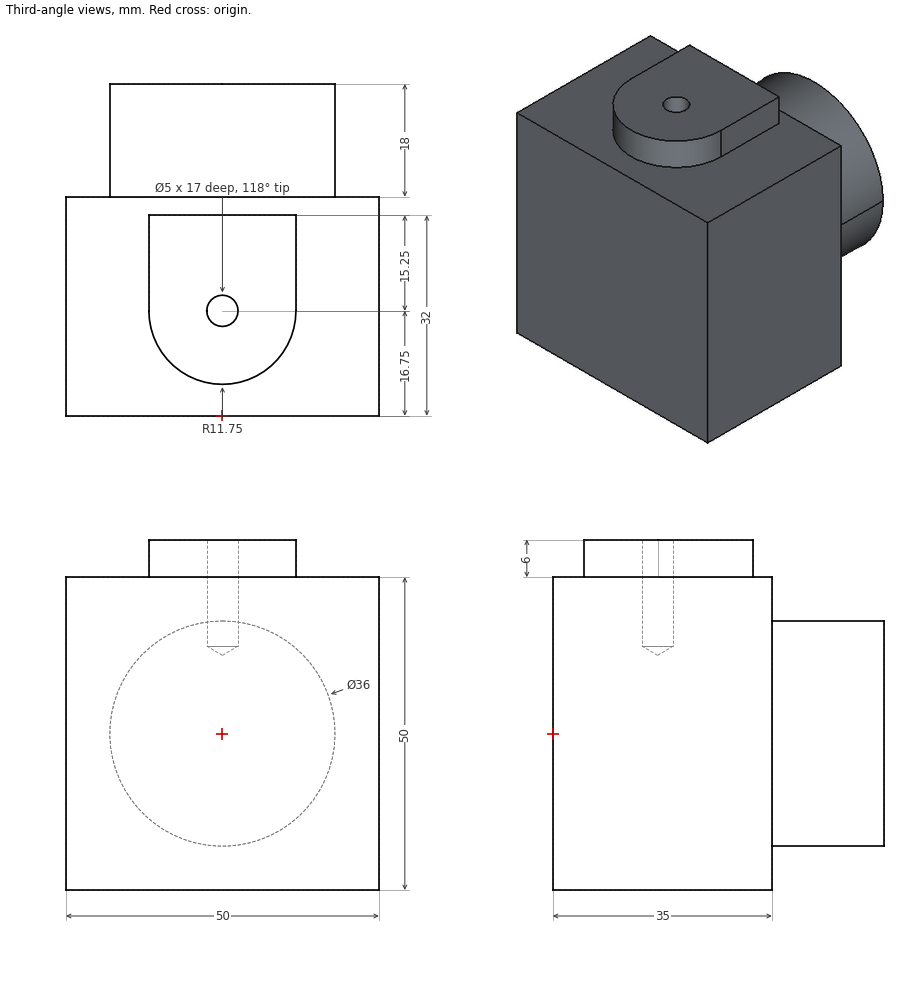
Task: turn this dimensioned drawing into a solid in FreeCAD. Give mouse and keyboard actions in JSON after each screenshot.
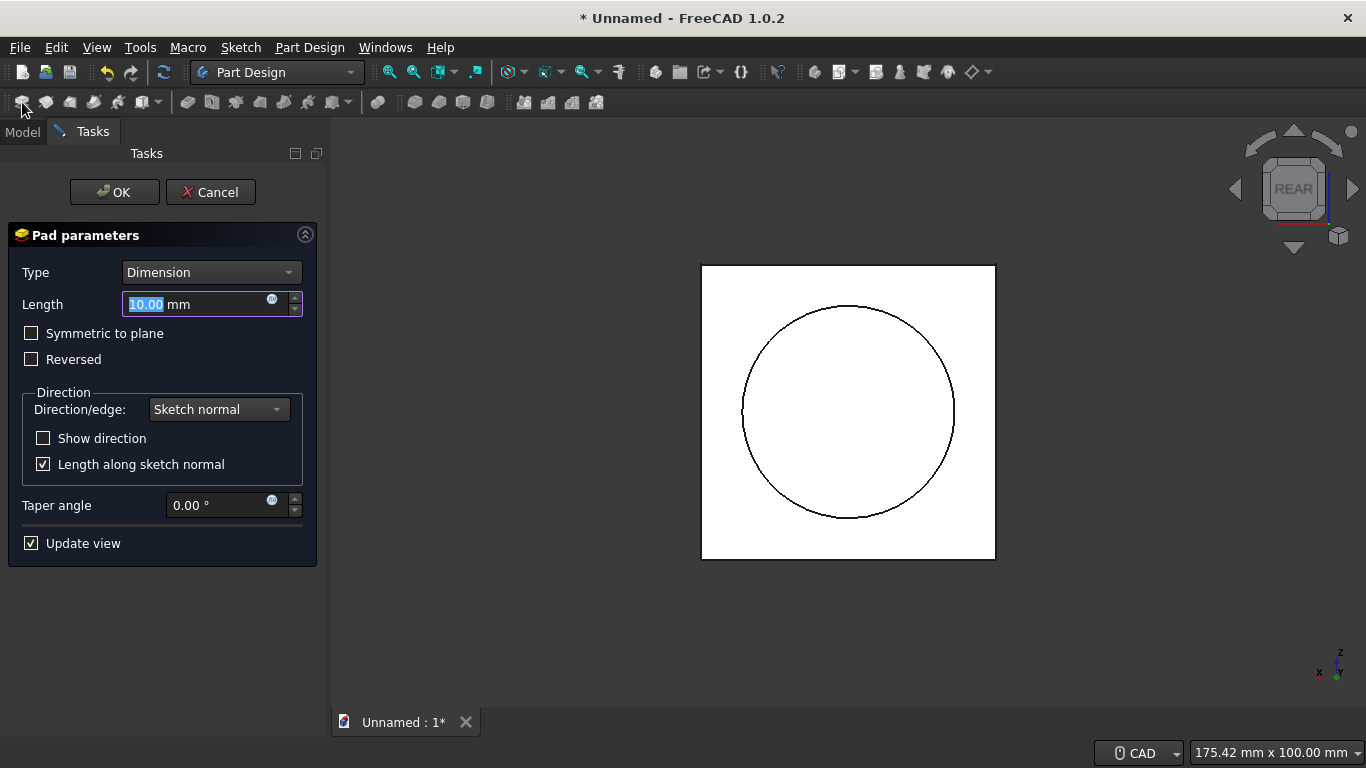
{"action": "type", "text": "18"}
{"action": "key", "text": "Tab"}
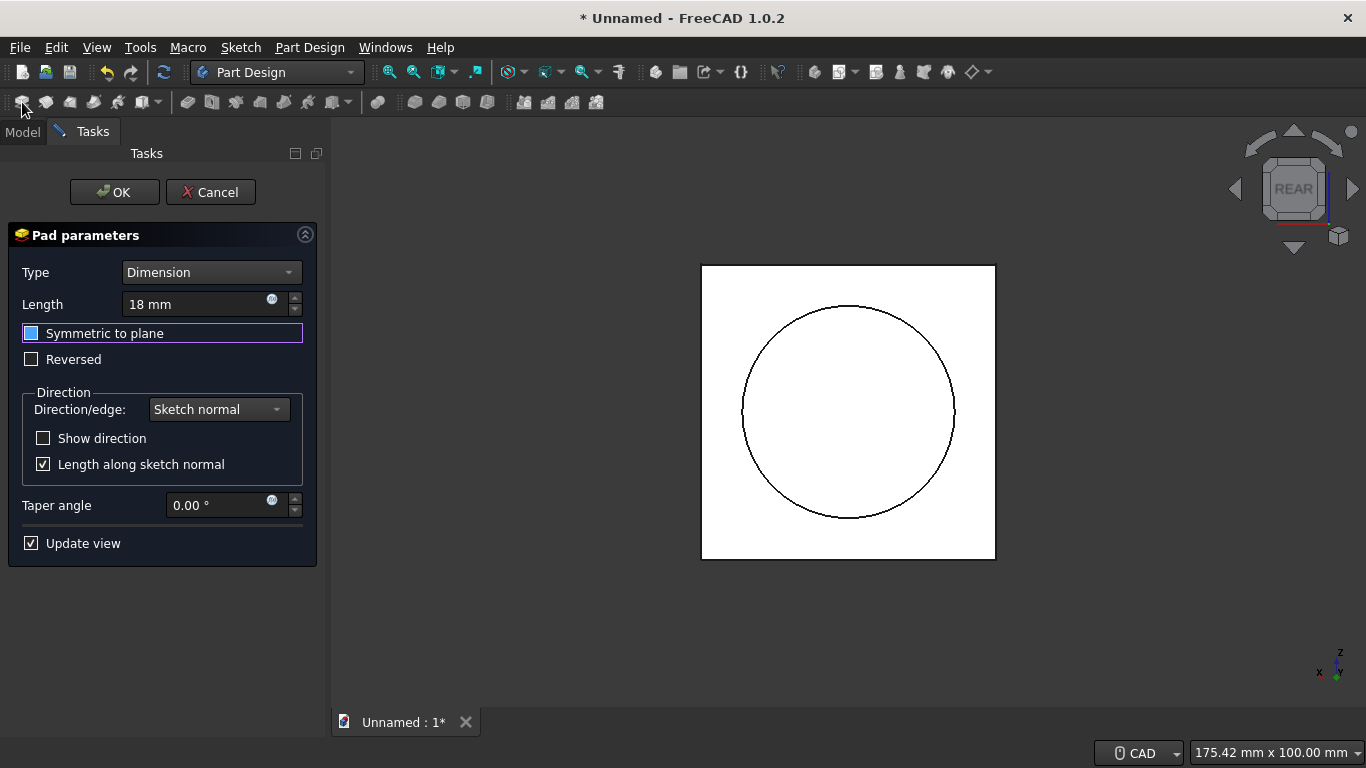
{"action": "left_click", "coordinate": [115, 192]}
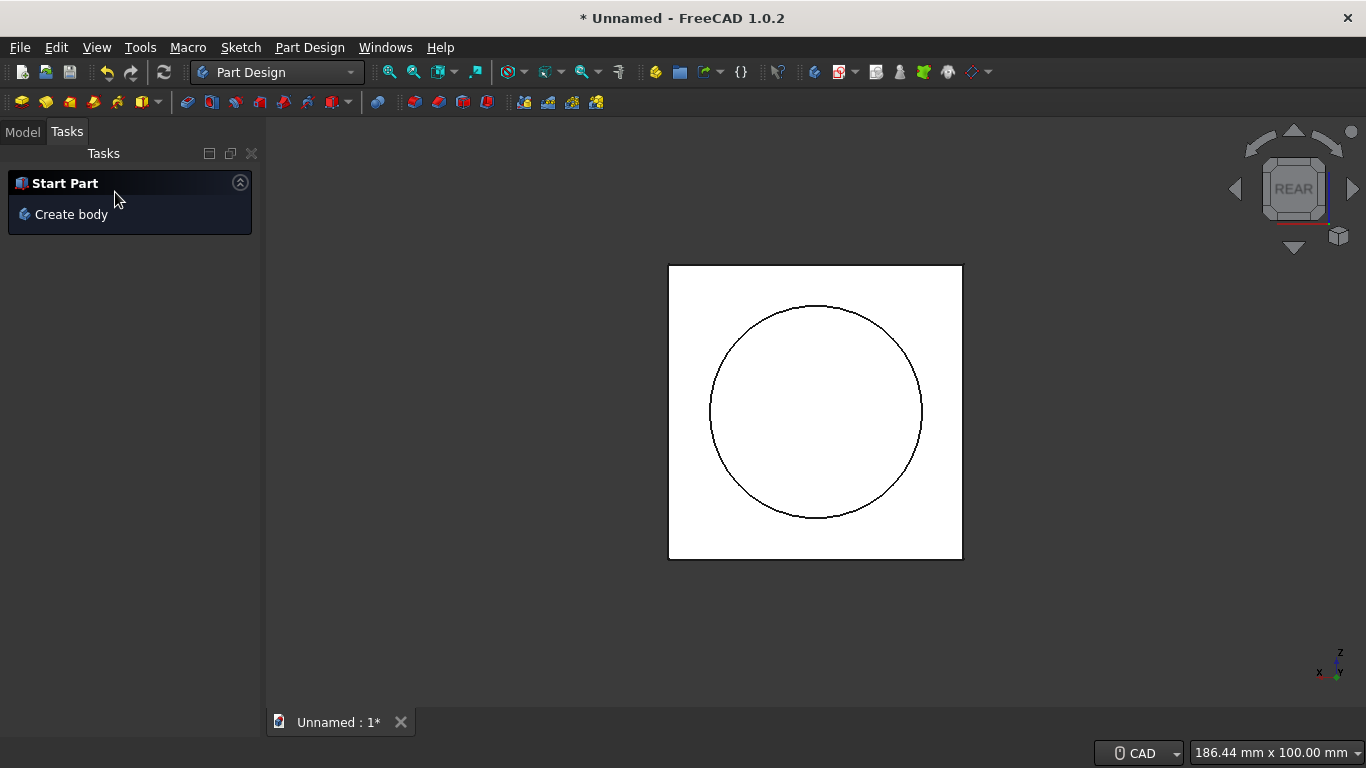
{"action": "key", "text": "0"}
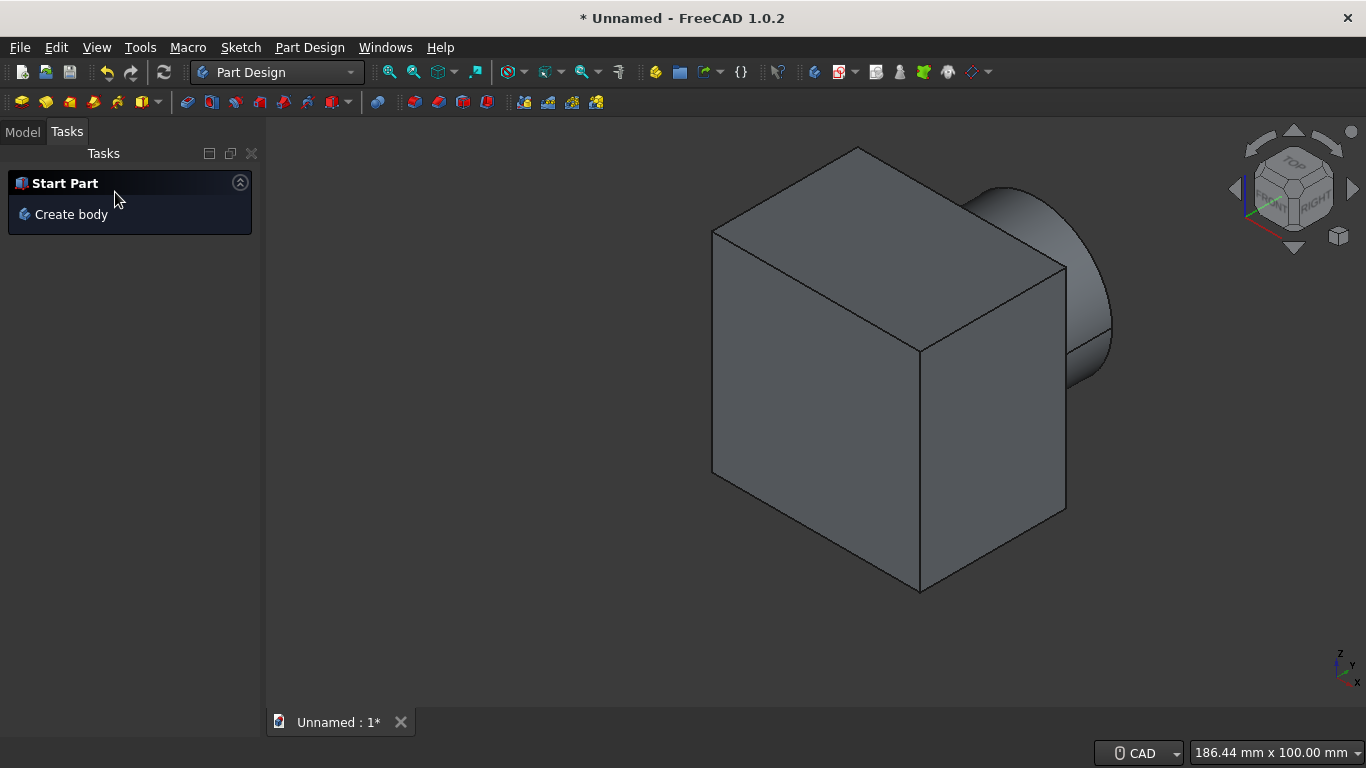
{"action": "key", "text": "v f"}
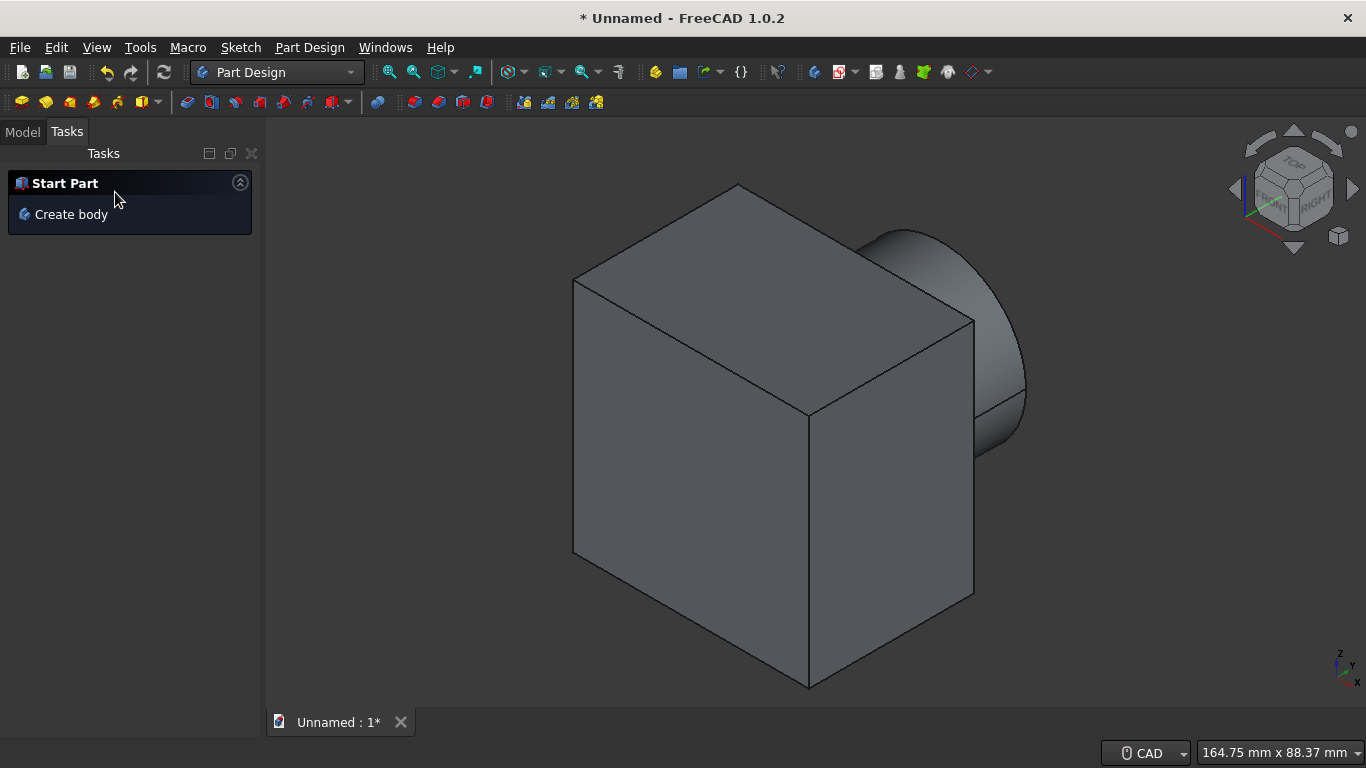
{"action": "left_click", "coordinate": [807, 319]}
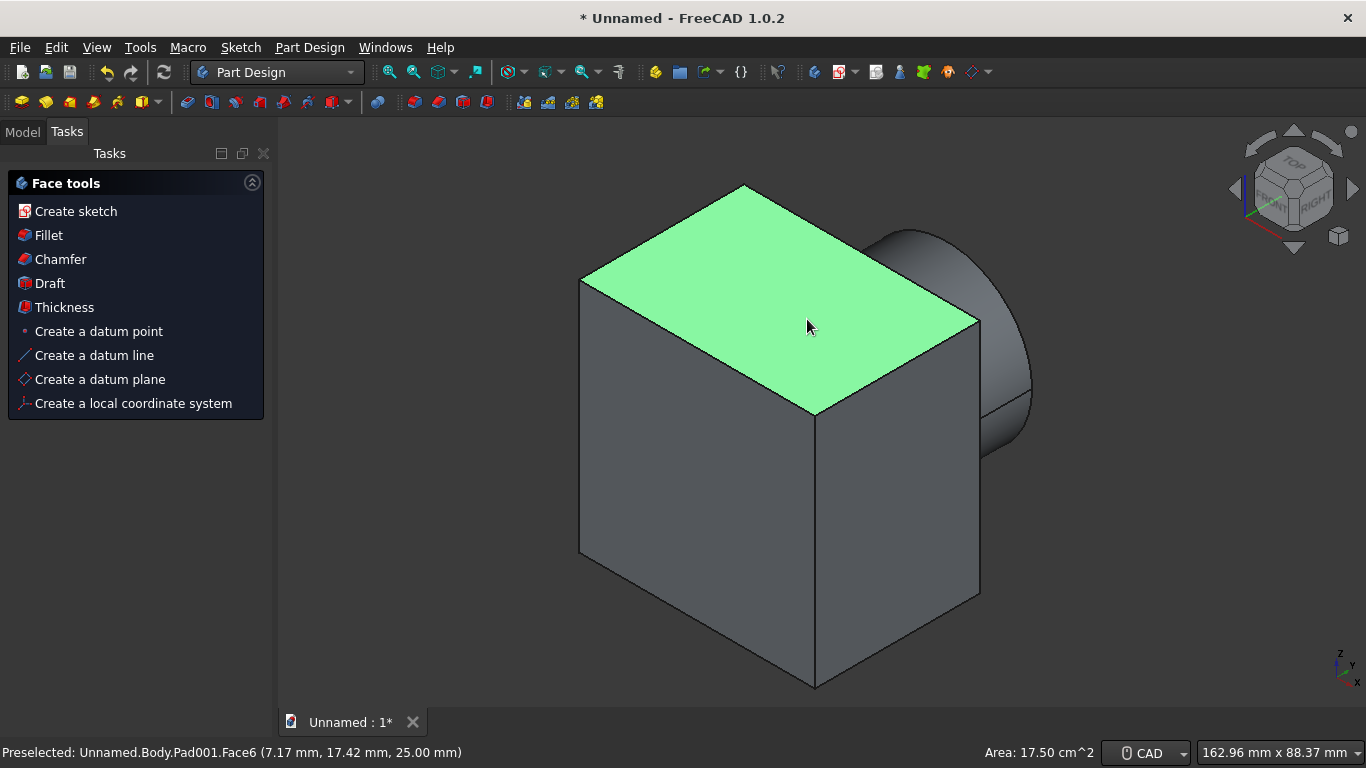
{"action": "left_click", "coordinate": [840, 72]}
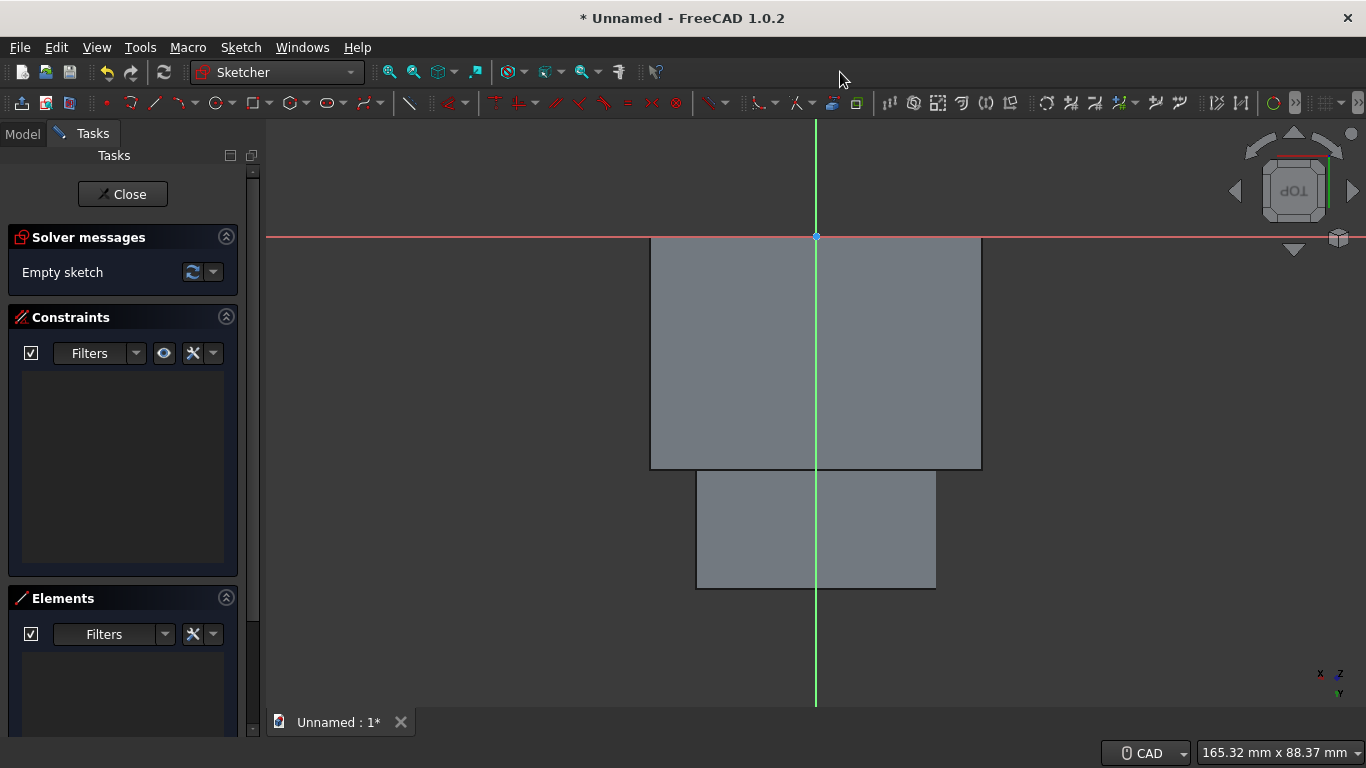
{"action": "scroll", "coordinate": [899, 258], "scroll_direction": "up", "scroll_amount": 3}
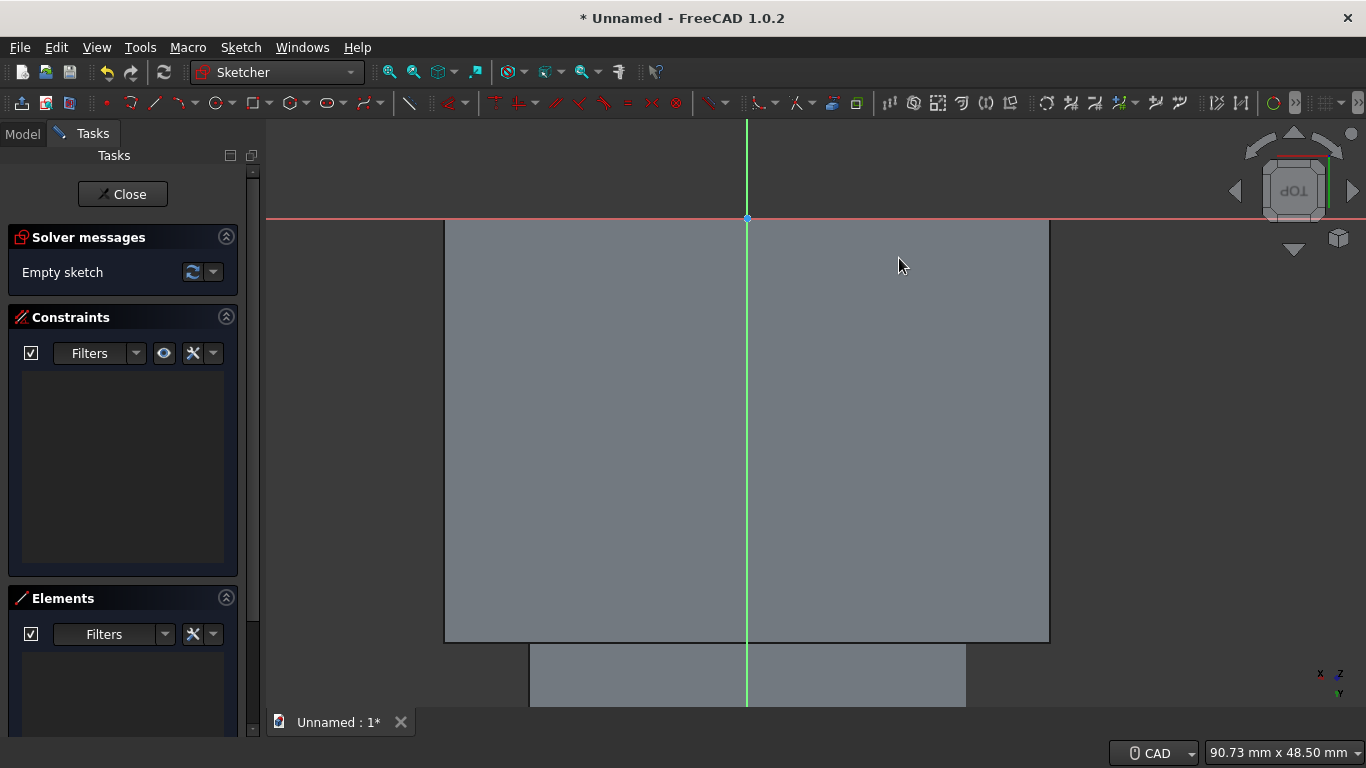
{"action": "left_click", "coordinate": [132, 104]}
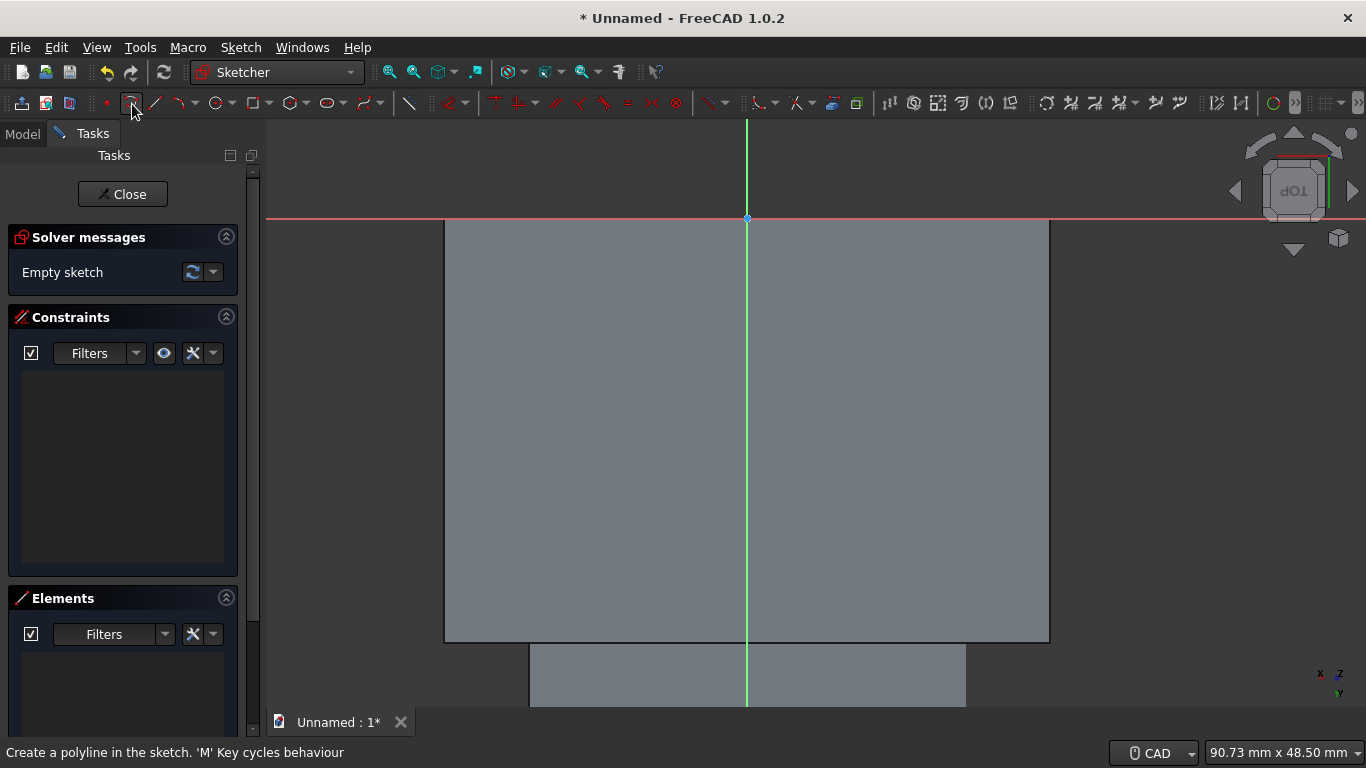
{"action": "left_click", "coordinate": [605, 422]}
{"action": "left_click", "coordinate": [605, 607]}
{"action": "left_click", "coordinate": [890, 607]}
{"action": "left_click", "coordinate": [890, 422]}
{"action": "right_click", "coordinate": [890, 422]}